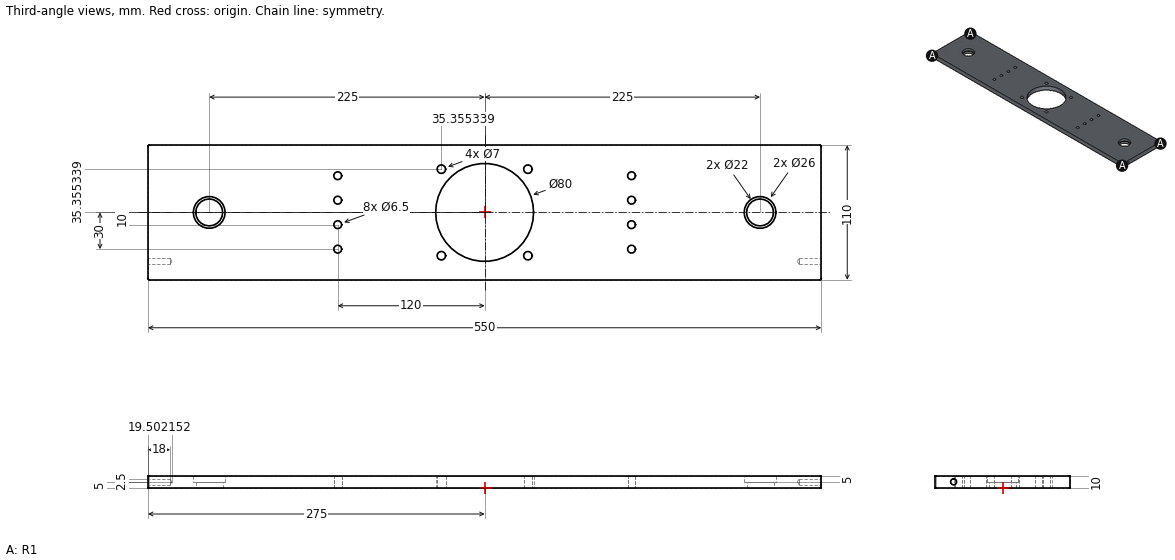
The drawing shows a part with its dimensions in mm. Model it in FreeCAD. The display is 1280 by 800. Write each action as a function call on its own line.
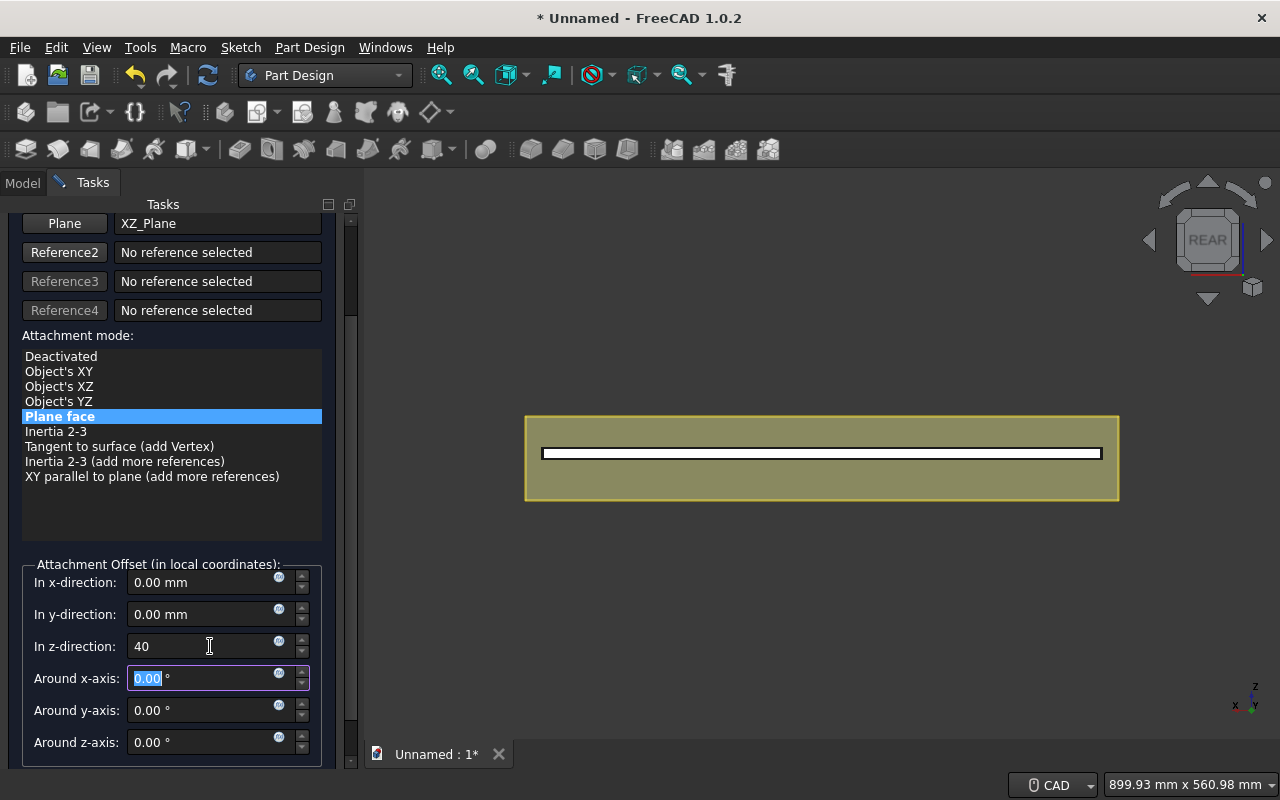
scroll(351, 491, up, 3)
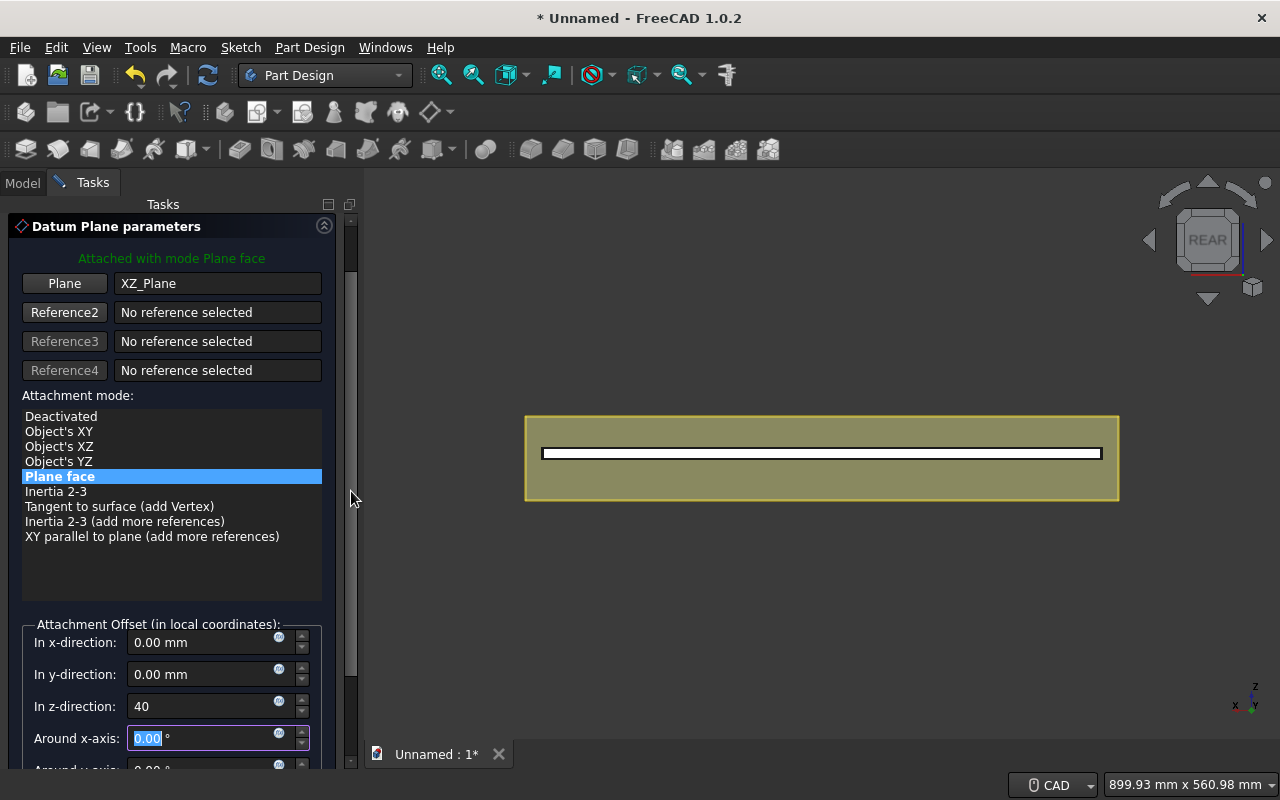
click(124, 243)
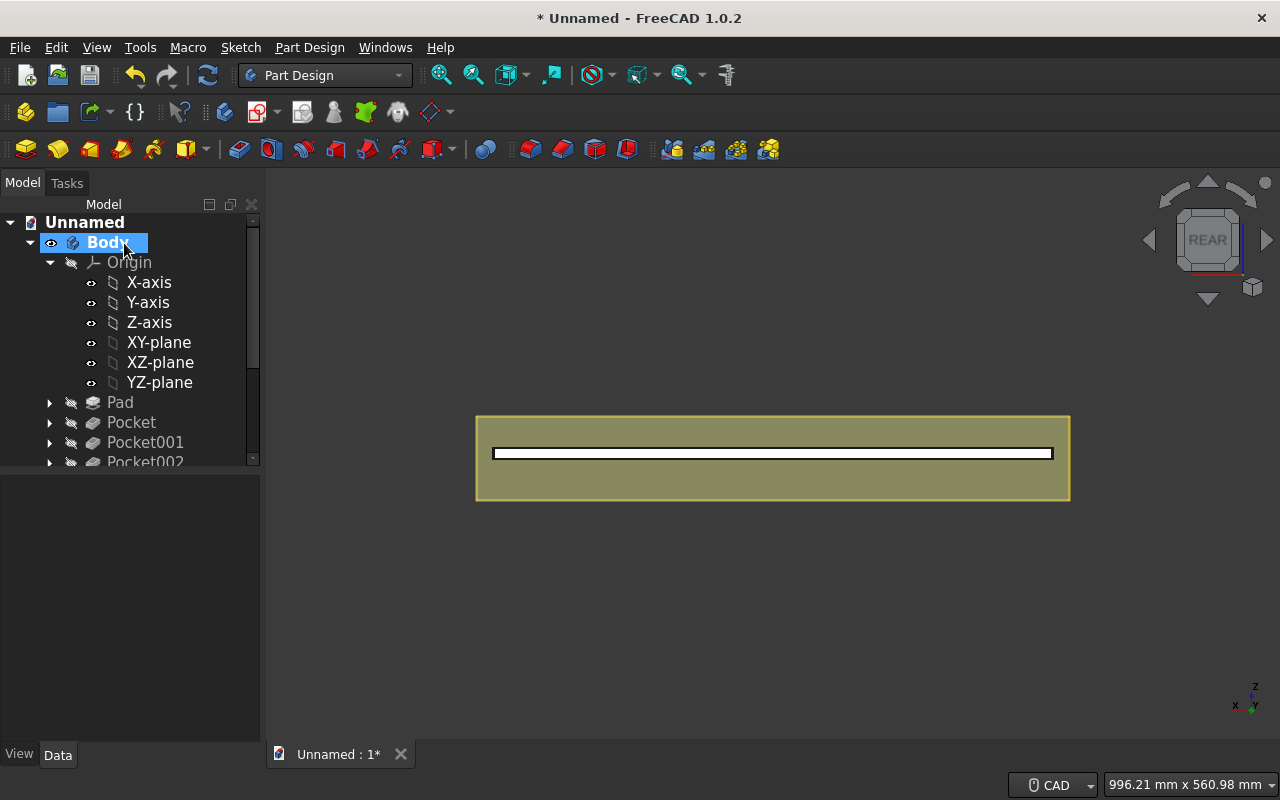
scroll(100, 338, down, 3)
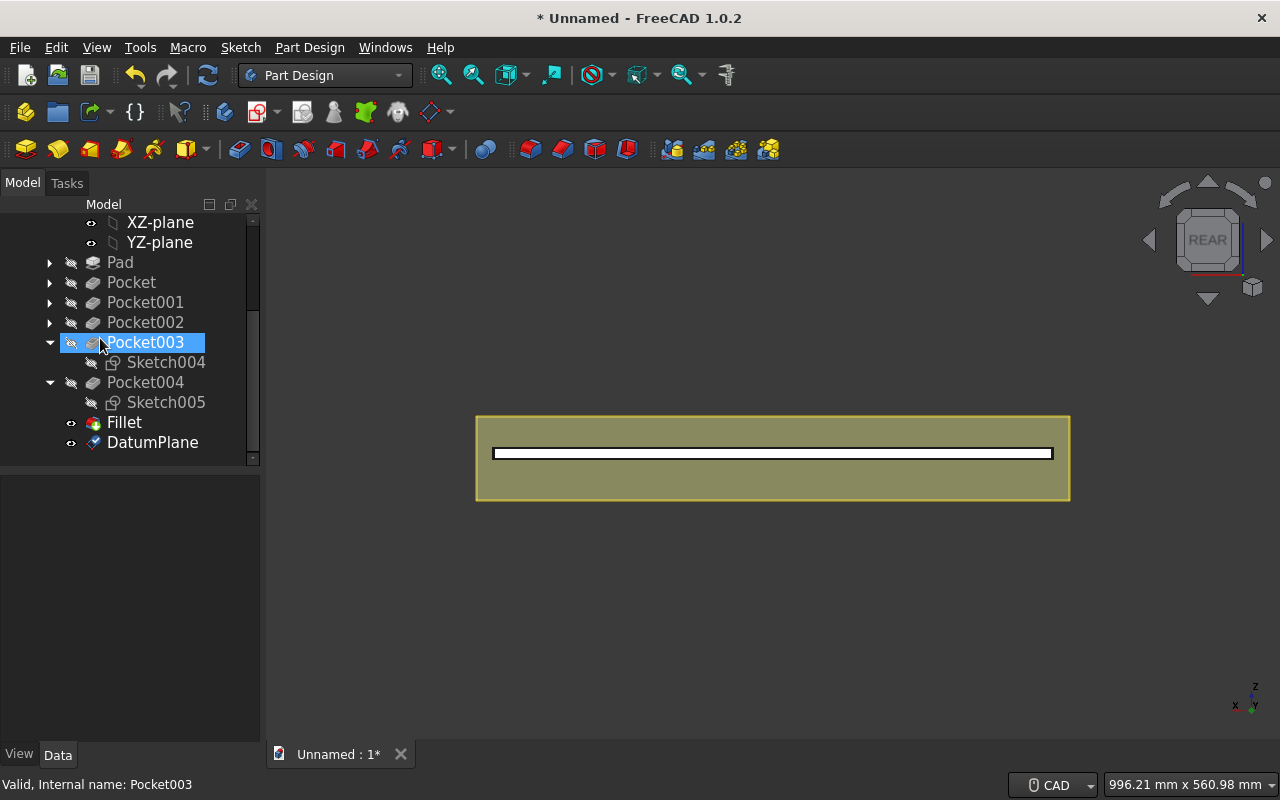
click(116, 443)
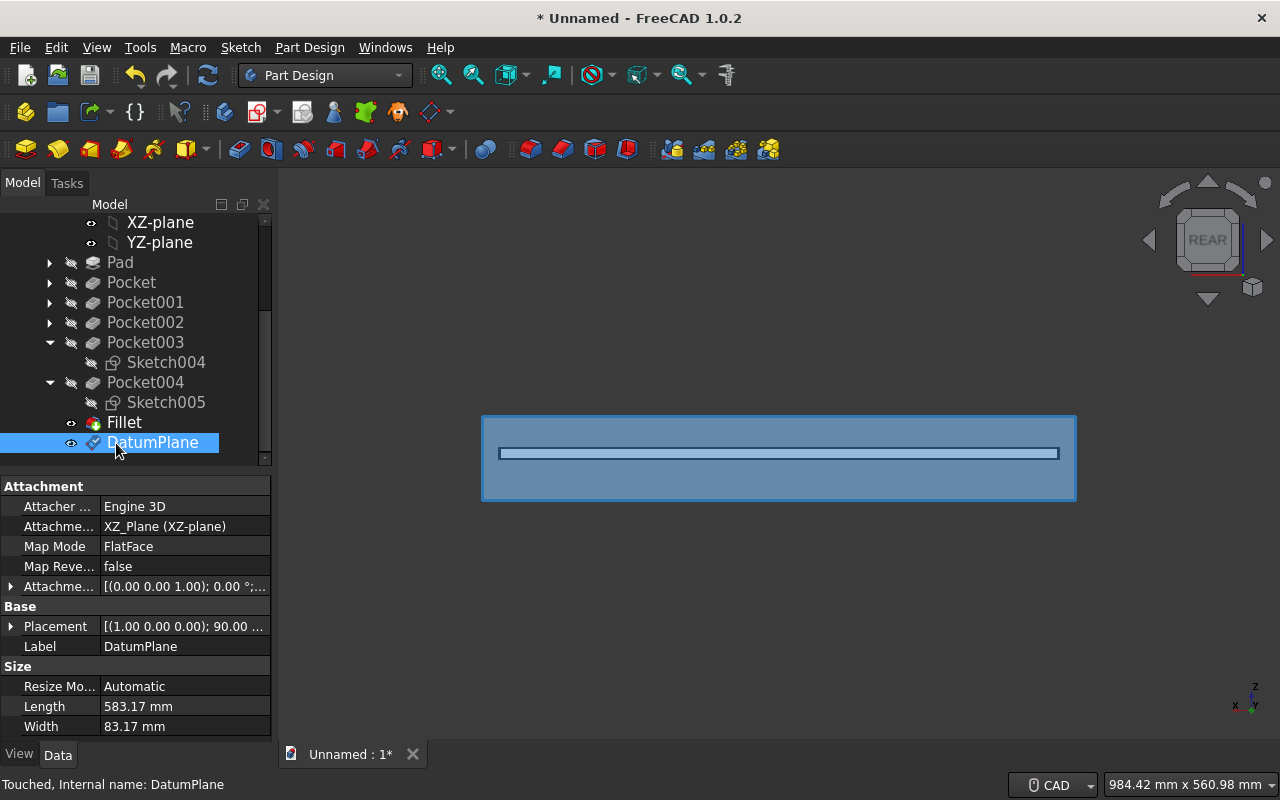
click(258, 112)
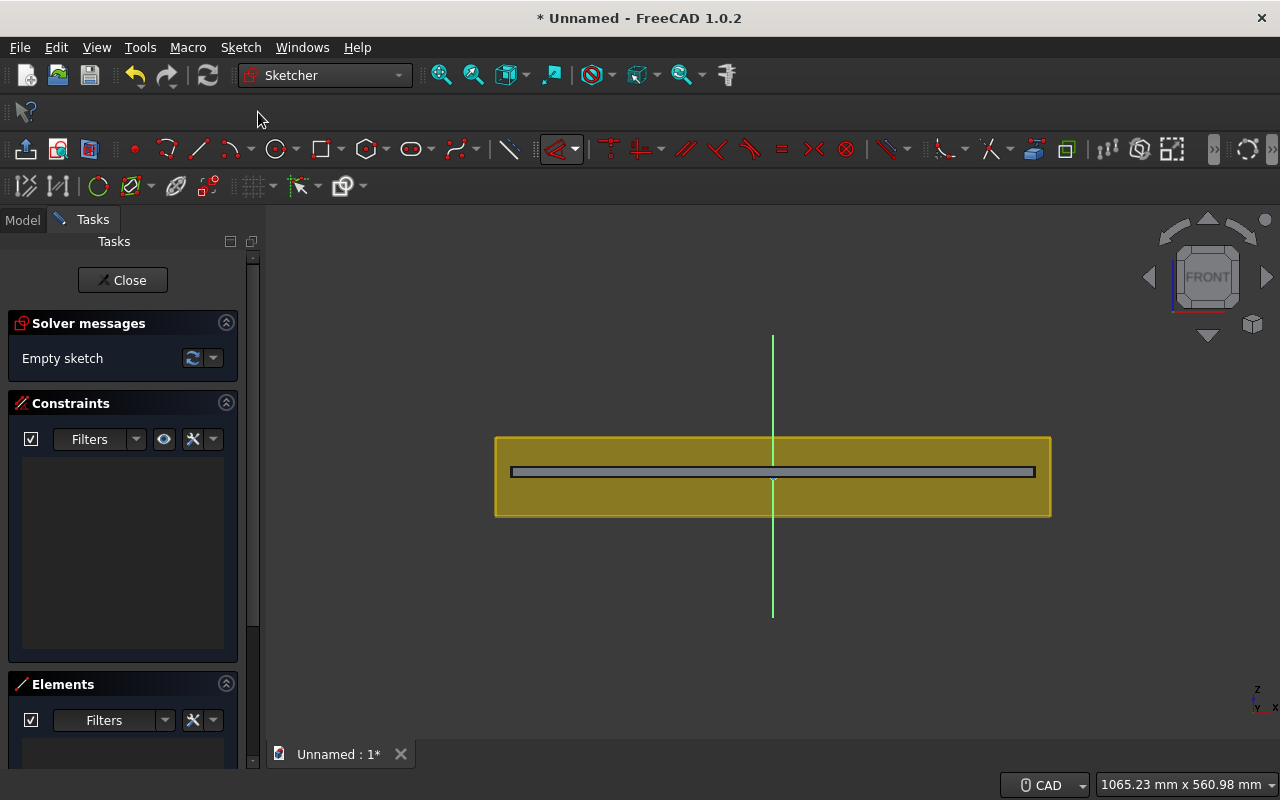
click(90, 150)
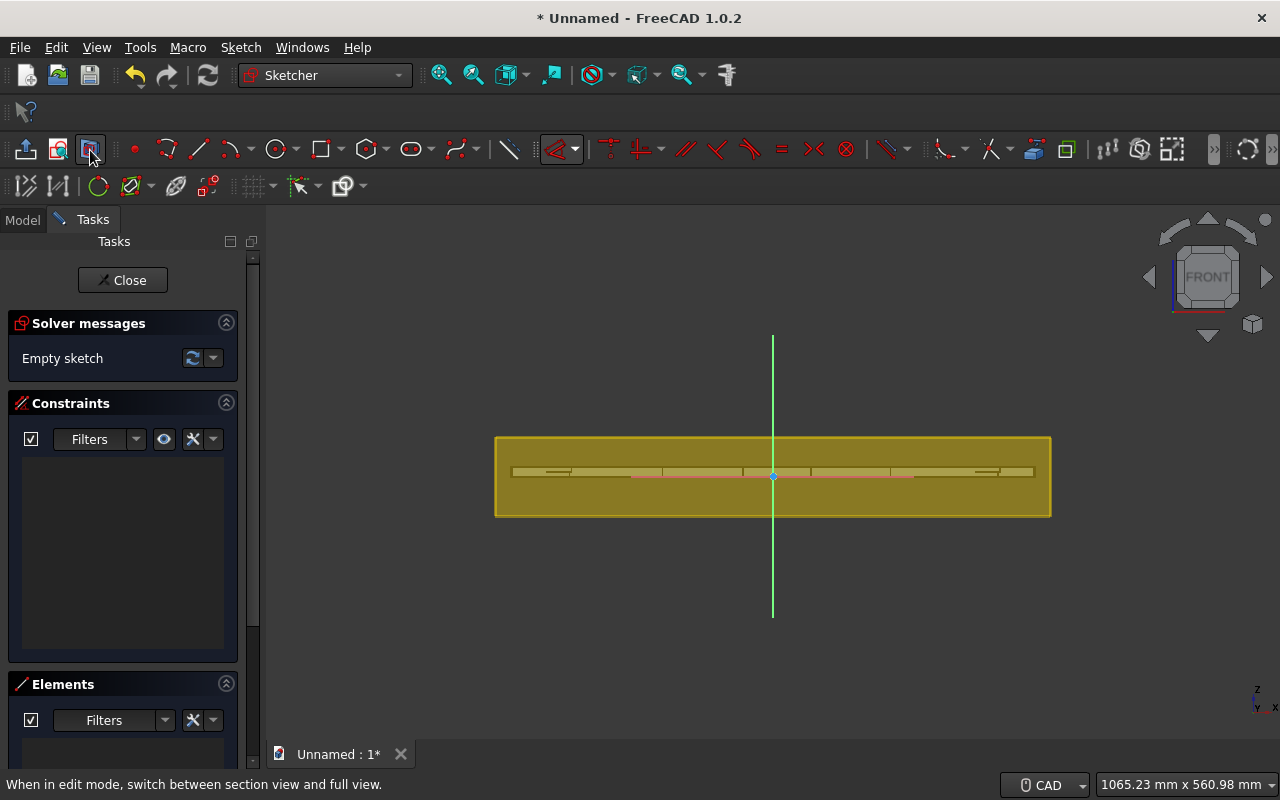
scroll(515, 471, up, 15)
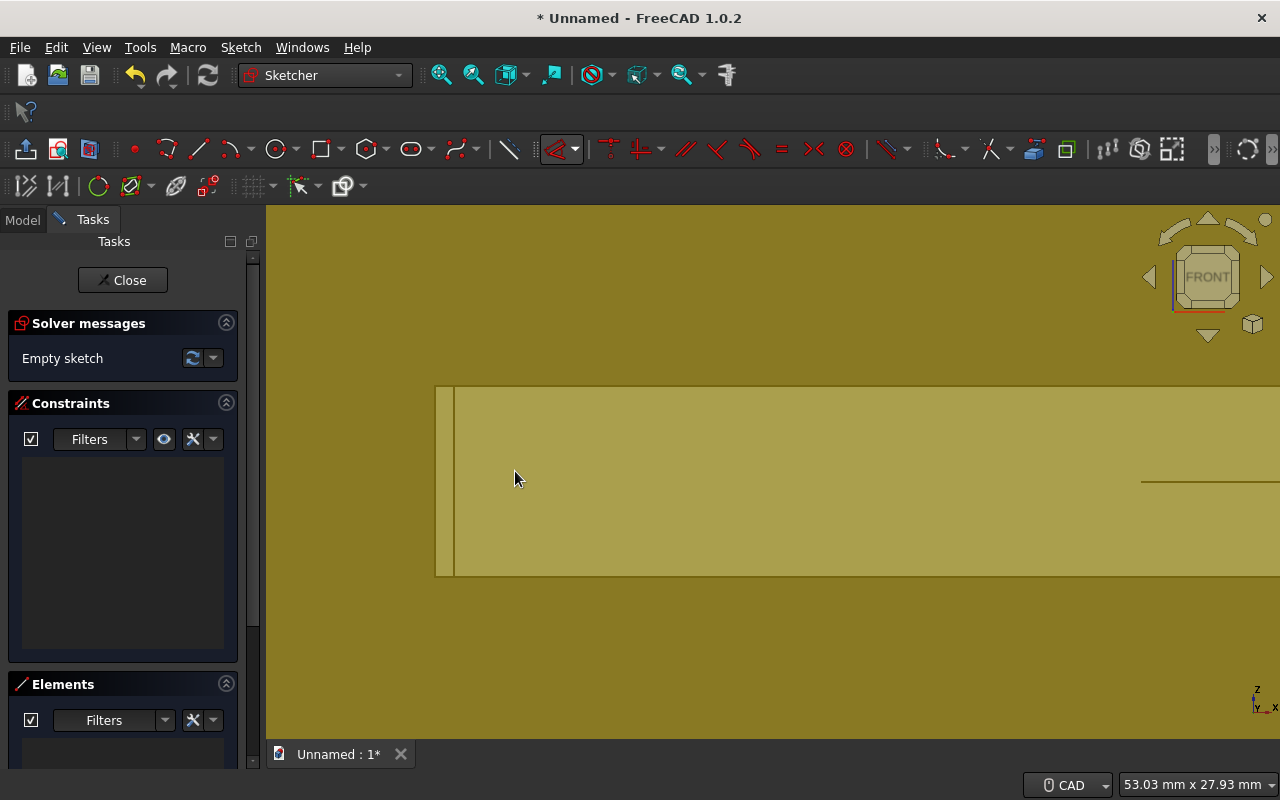
key(g)
key(m)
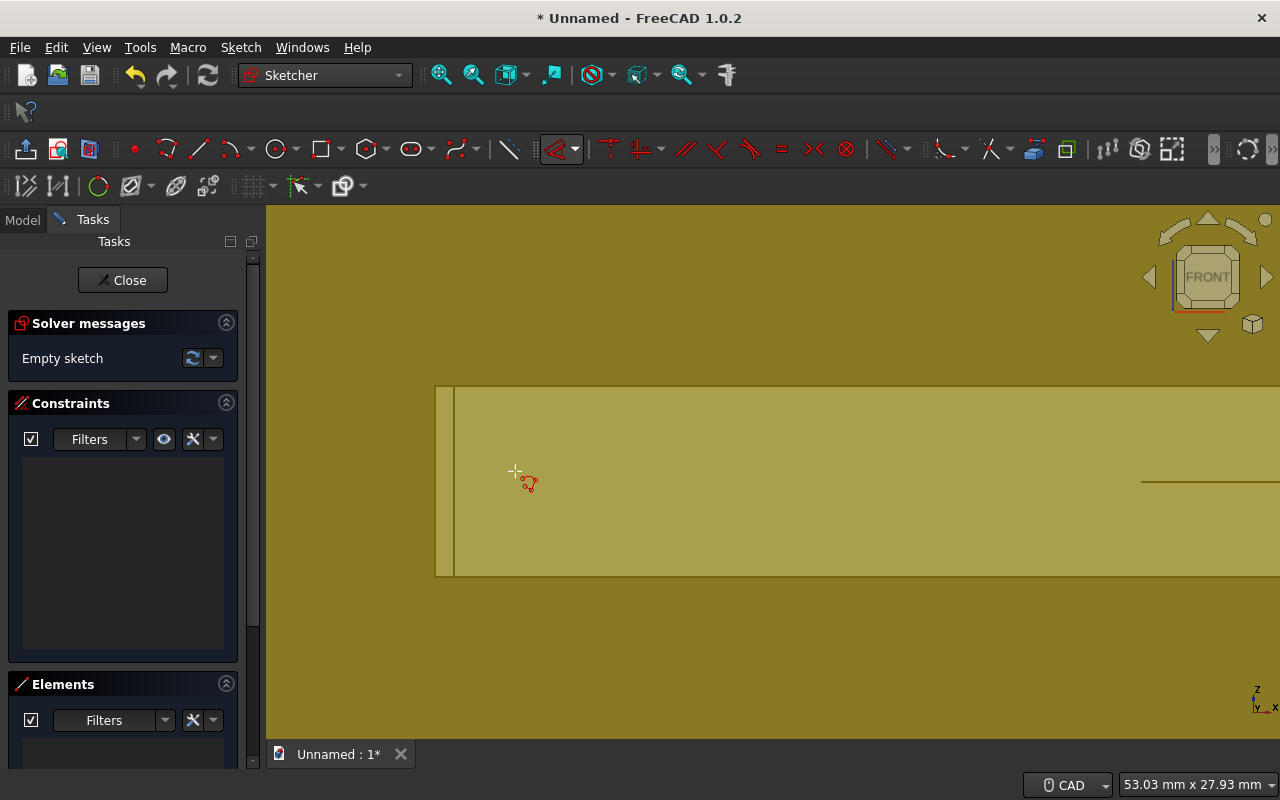
click(807, 482)
click(435, 482)
click(435, 434)
click(779, 434)
click(807, 483)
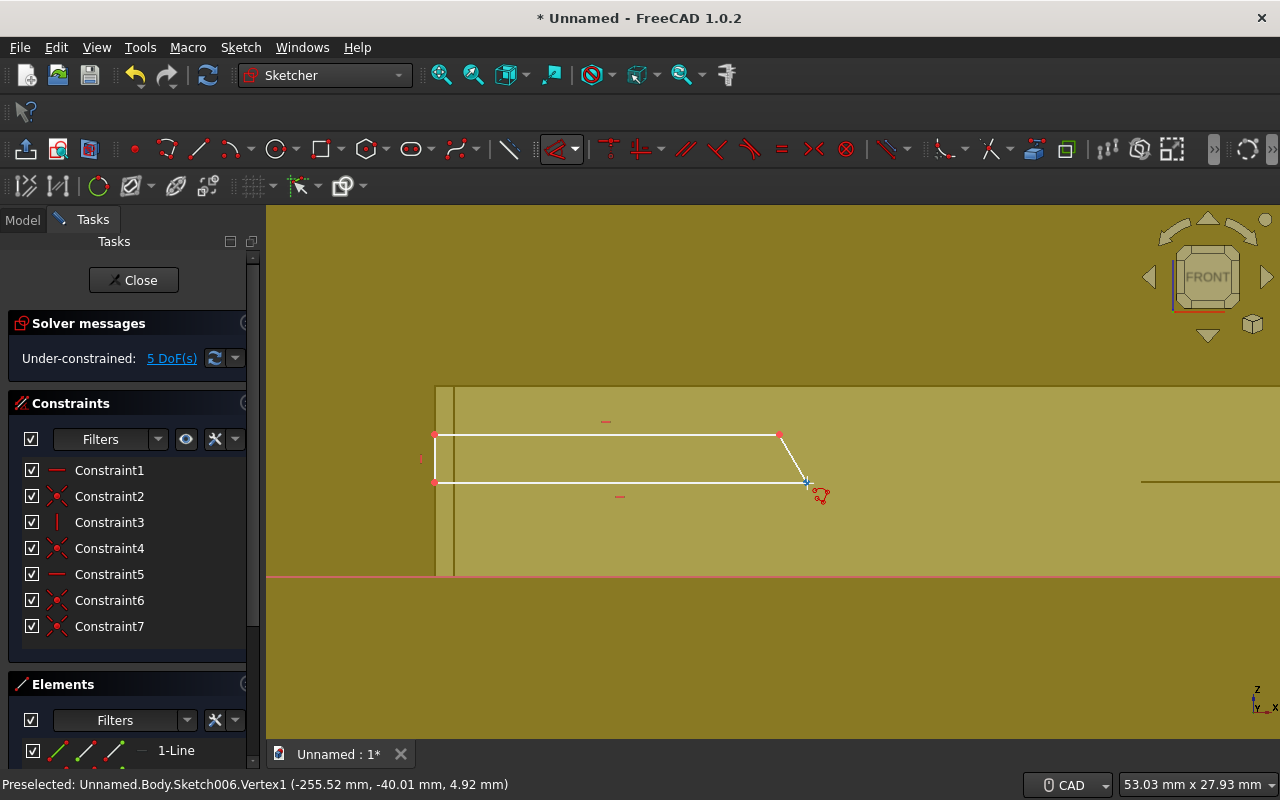
click(200, 150)